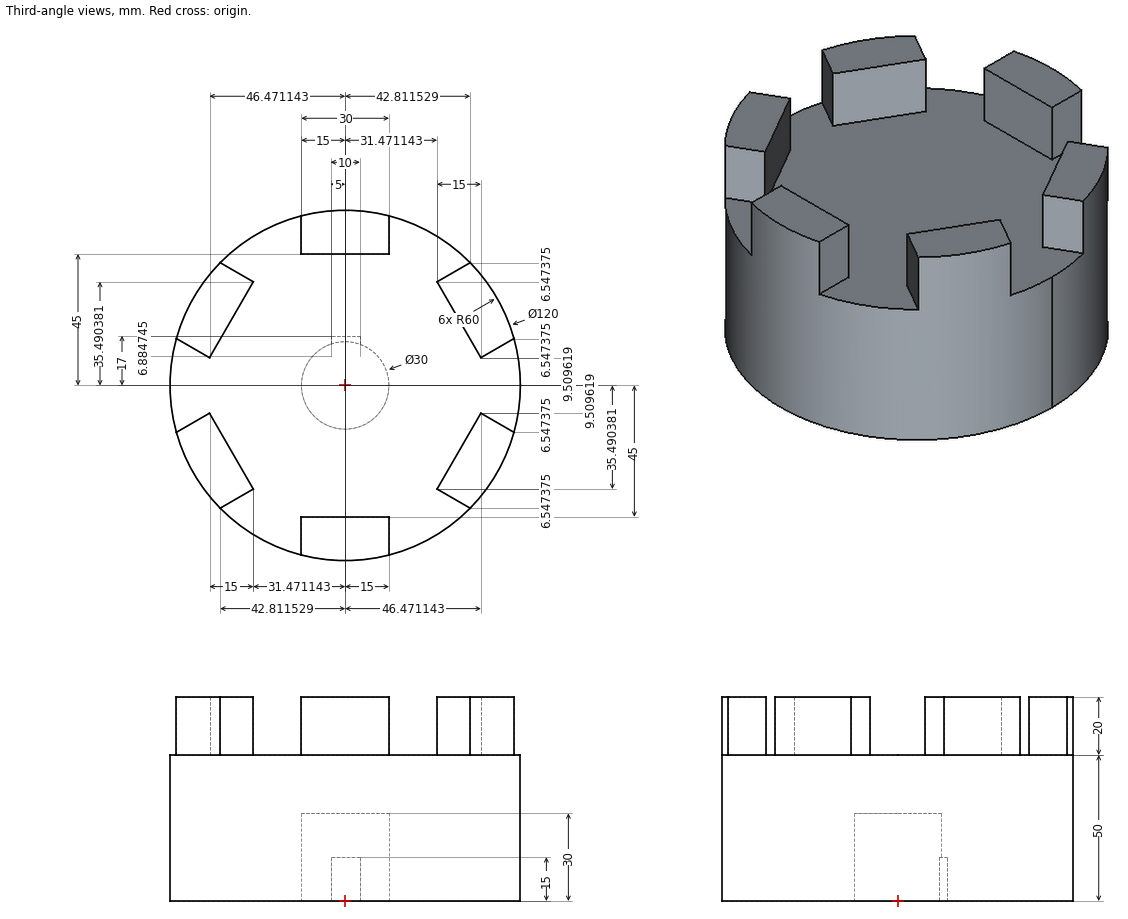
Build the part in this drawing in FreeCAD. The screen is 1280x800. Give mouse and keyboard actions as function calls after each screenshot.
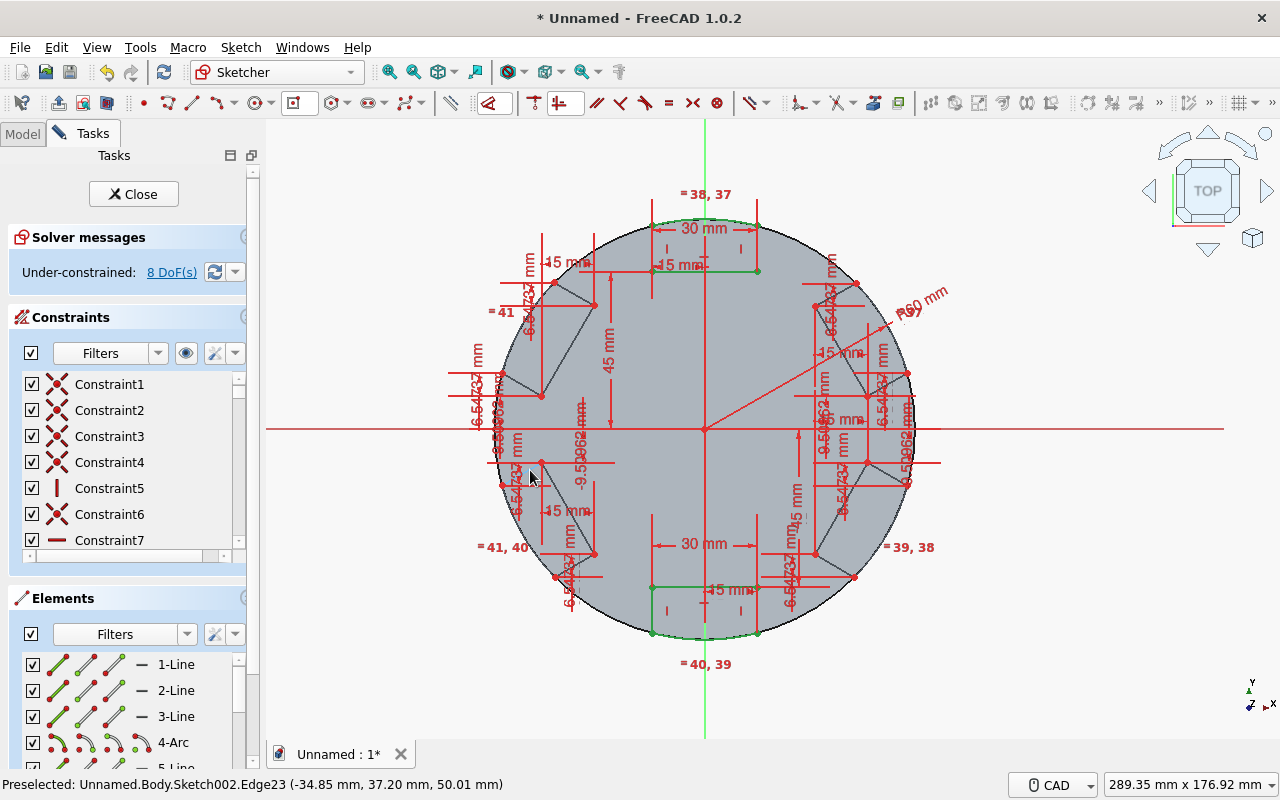
click(856, 284)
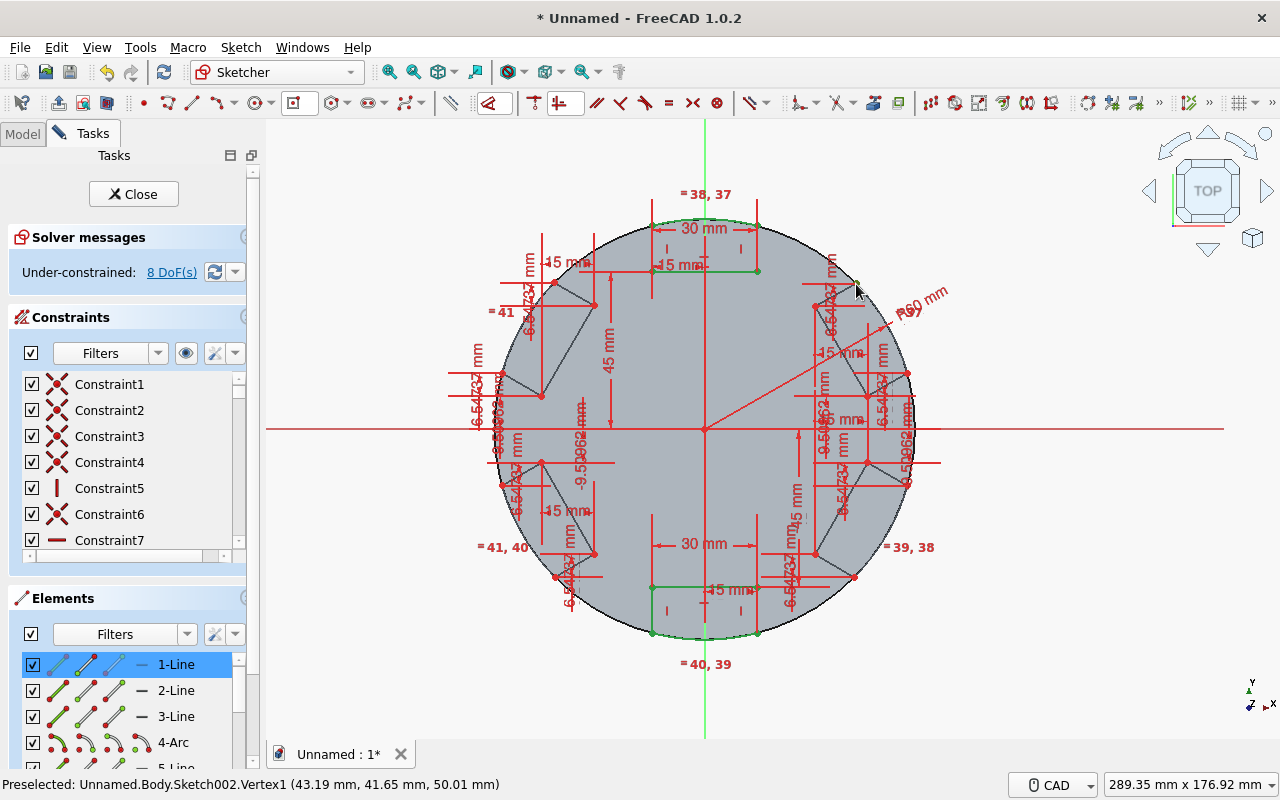
click(506, 104)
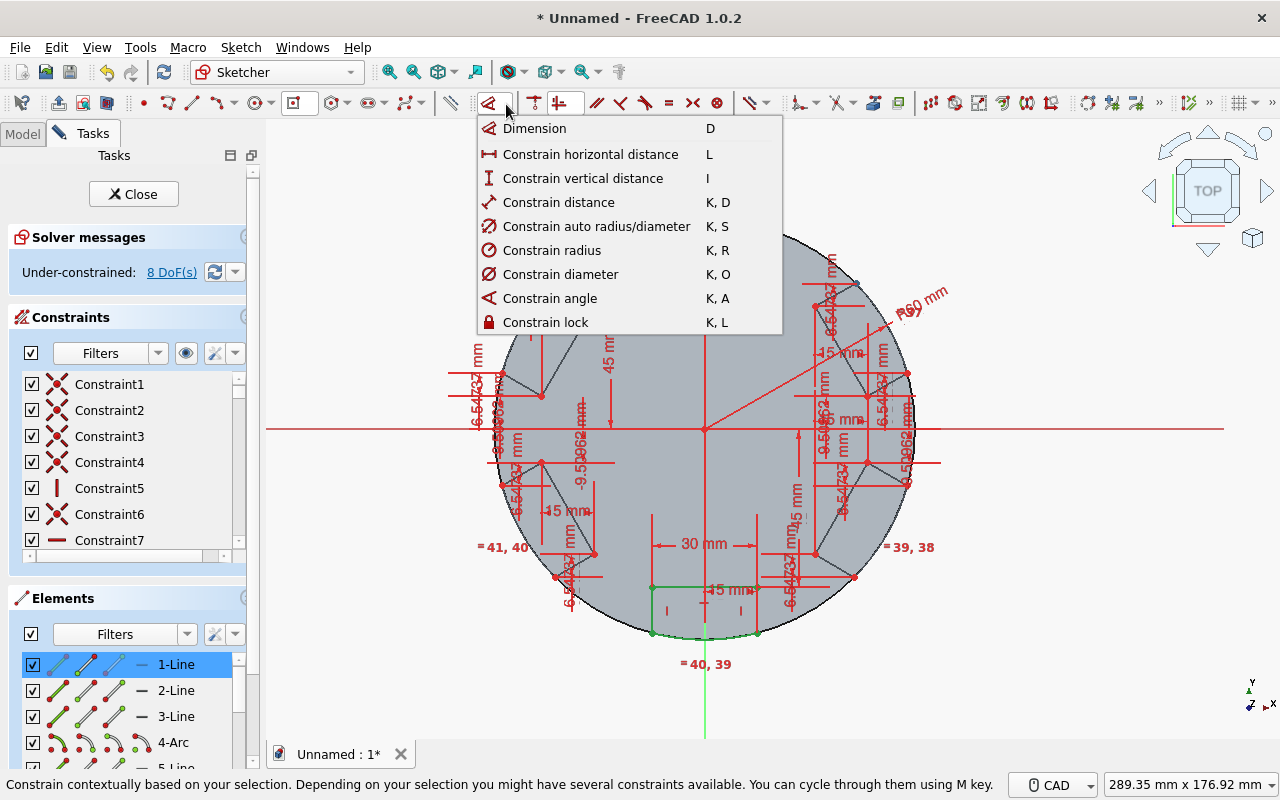
click(630, 154)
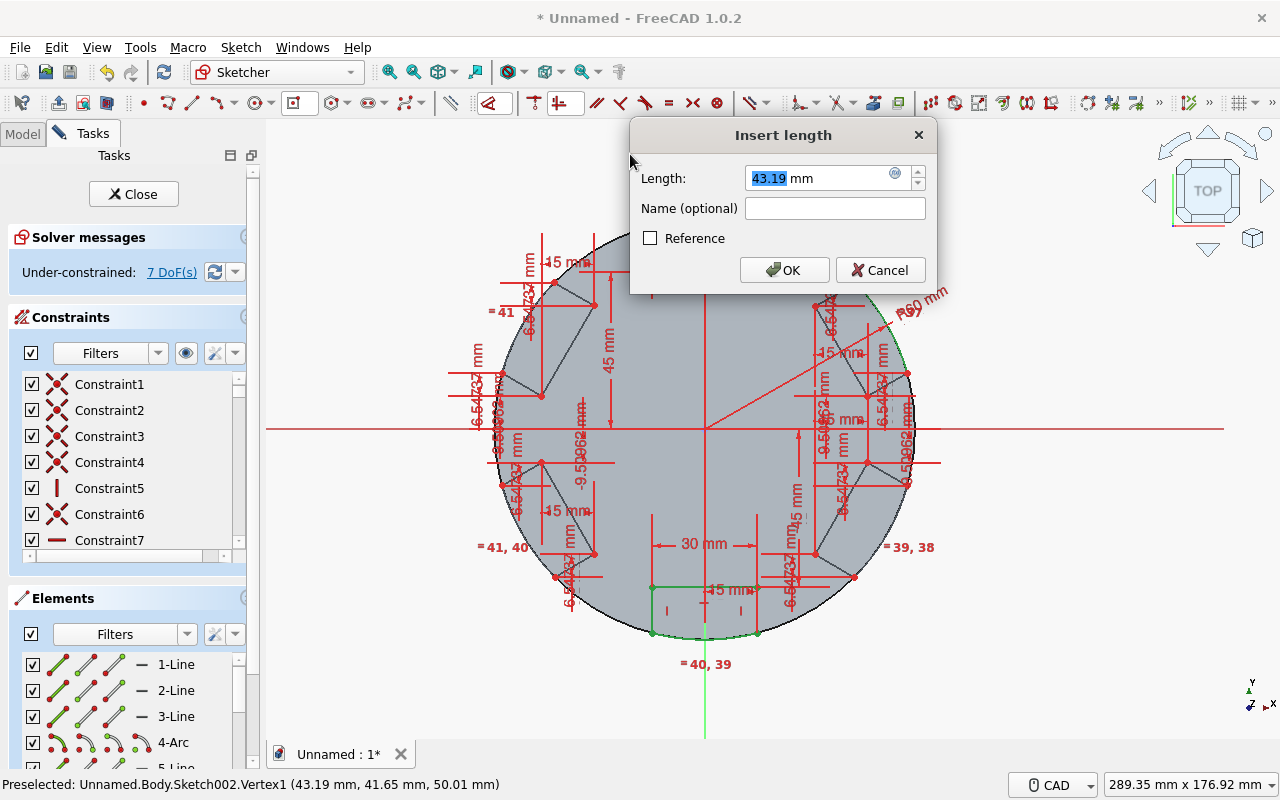
text(42.811529)
key(Return)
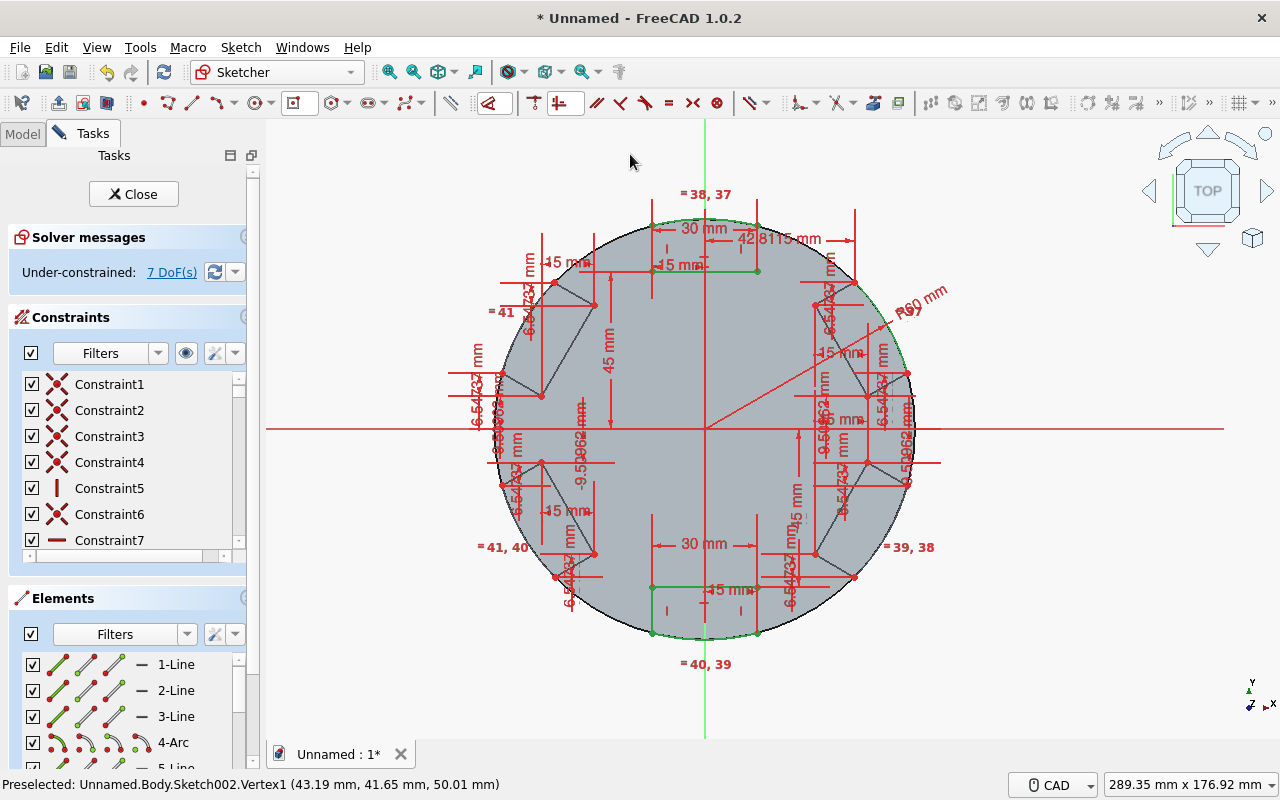
click(815, 305)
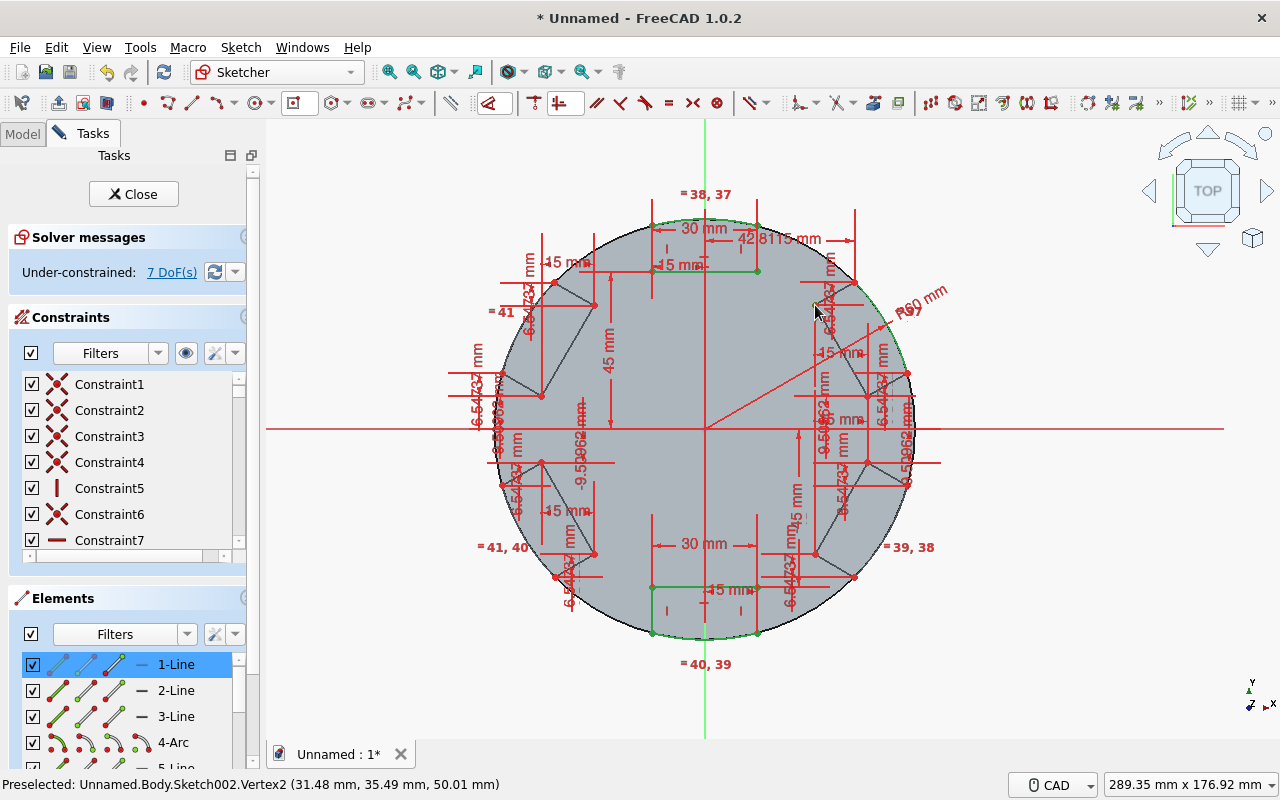
click(506, 104)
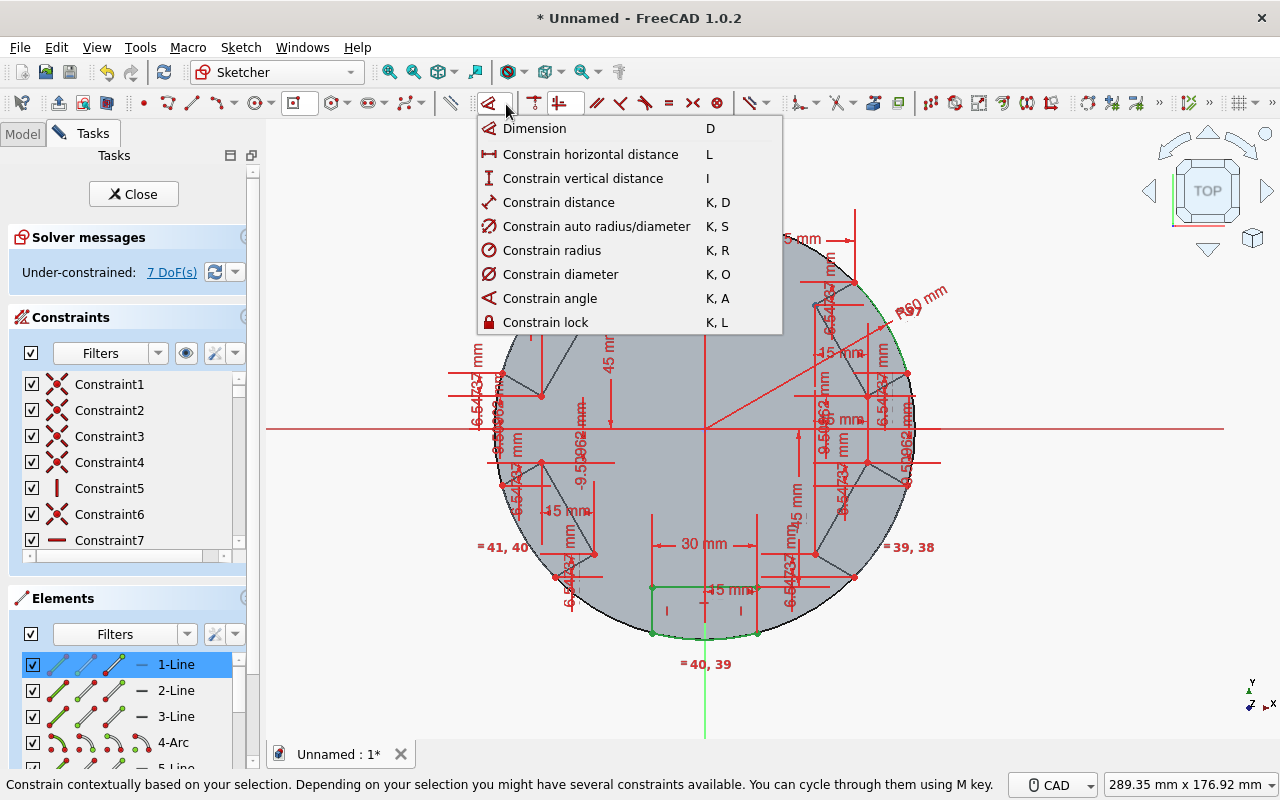
click(630, 154)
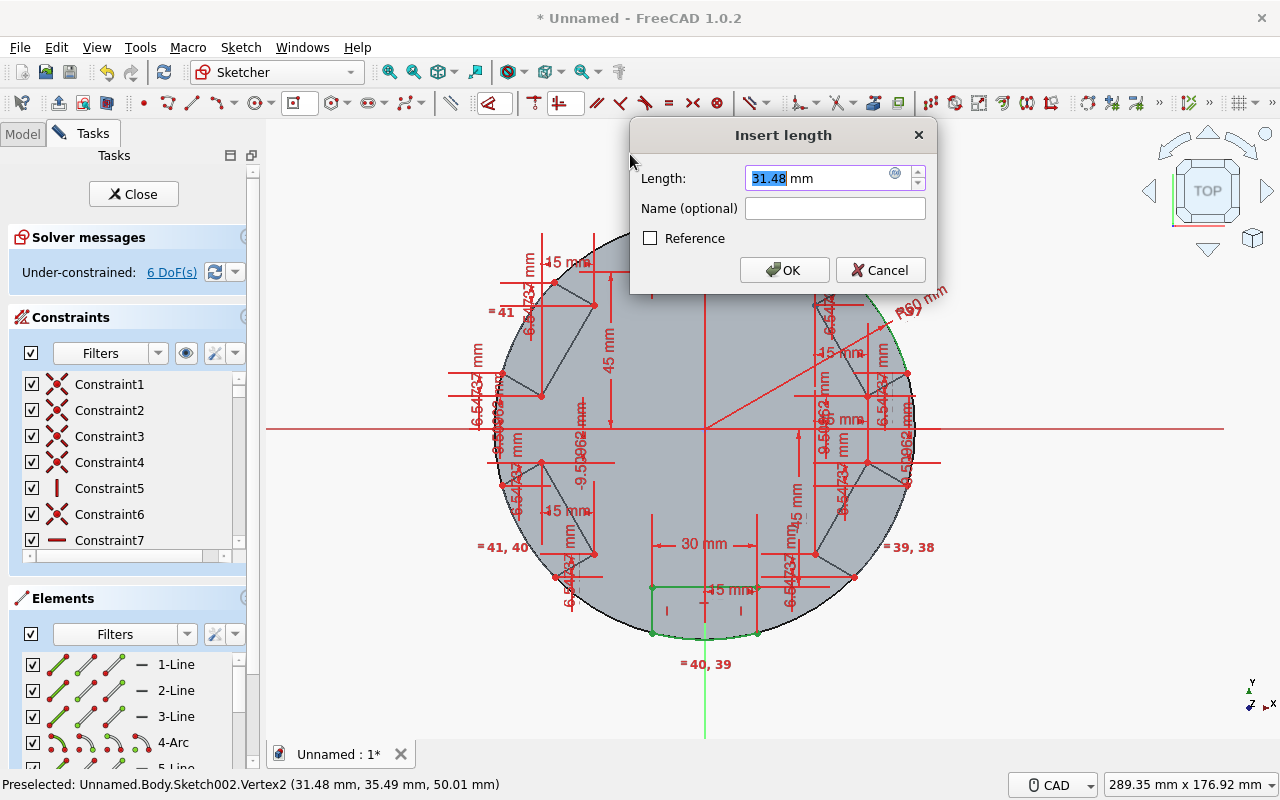
text(31.471143)
key(Return)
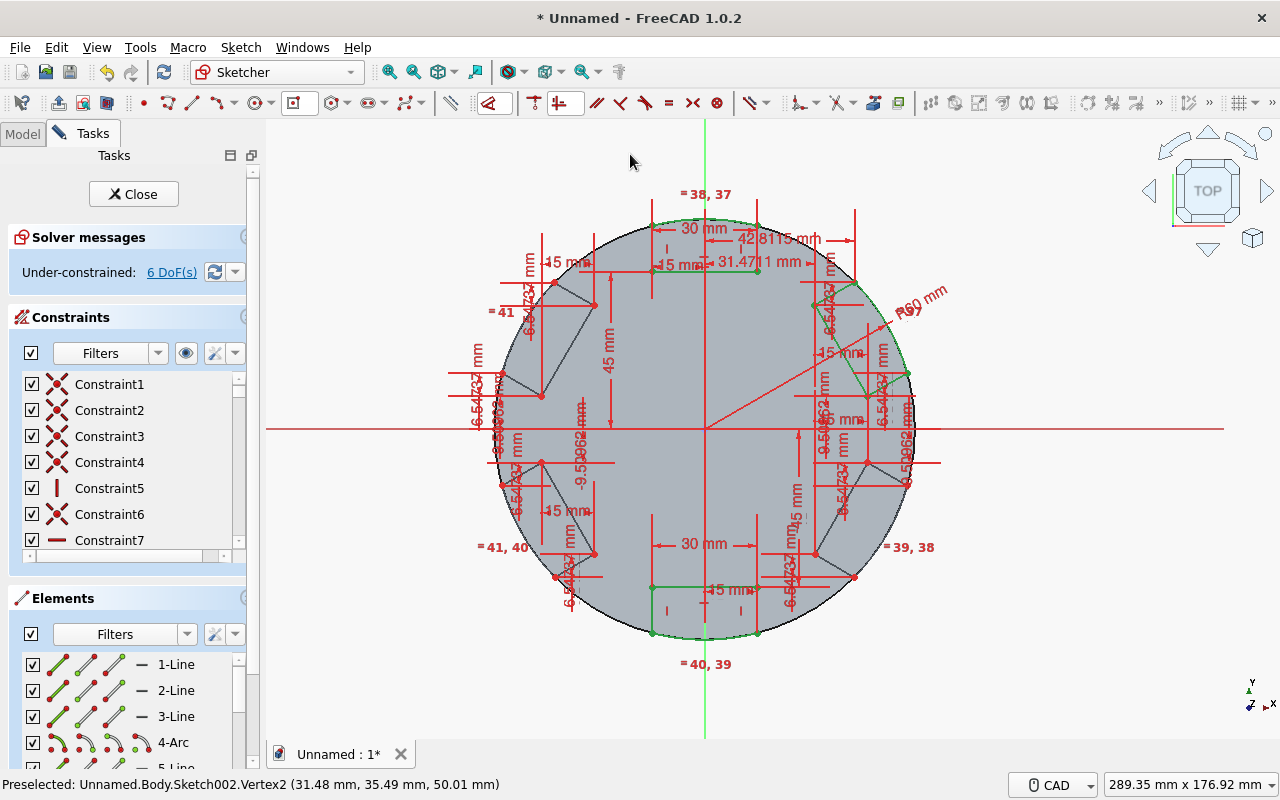
click(868, 463)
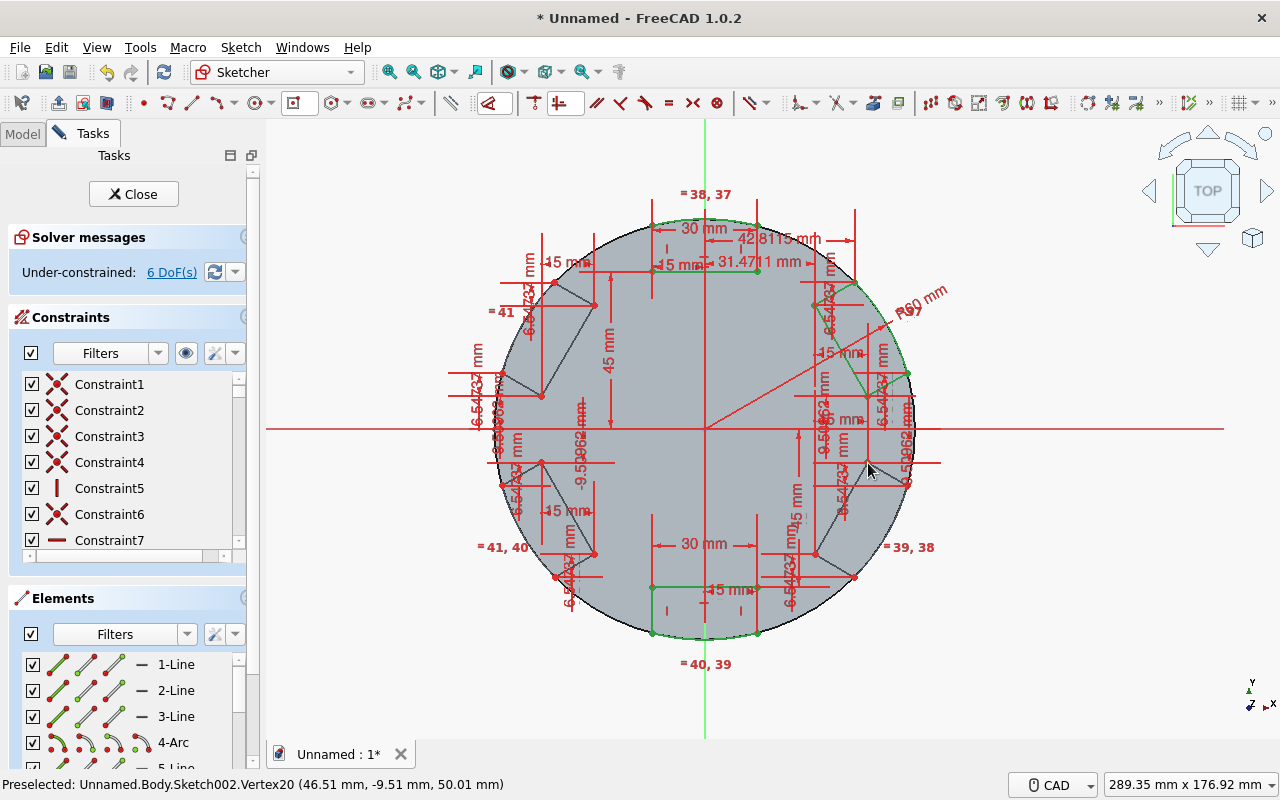
key(l)